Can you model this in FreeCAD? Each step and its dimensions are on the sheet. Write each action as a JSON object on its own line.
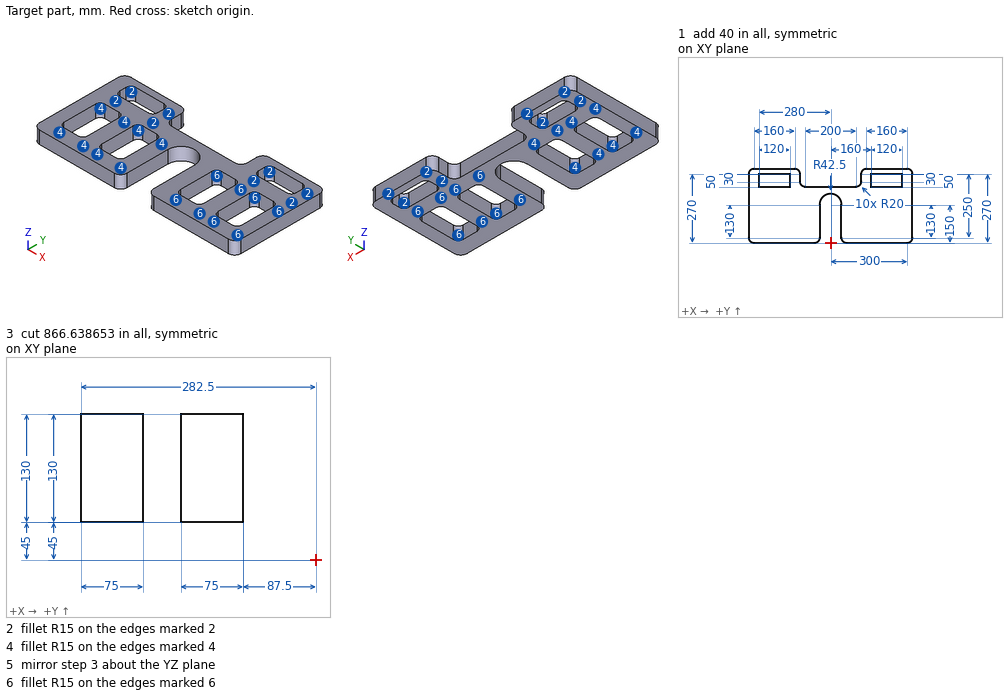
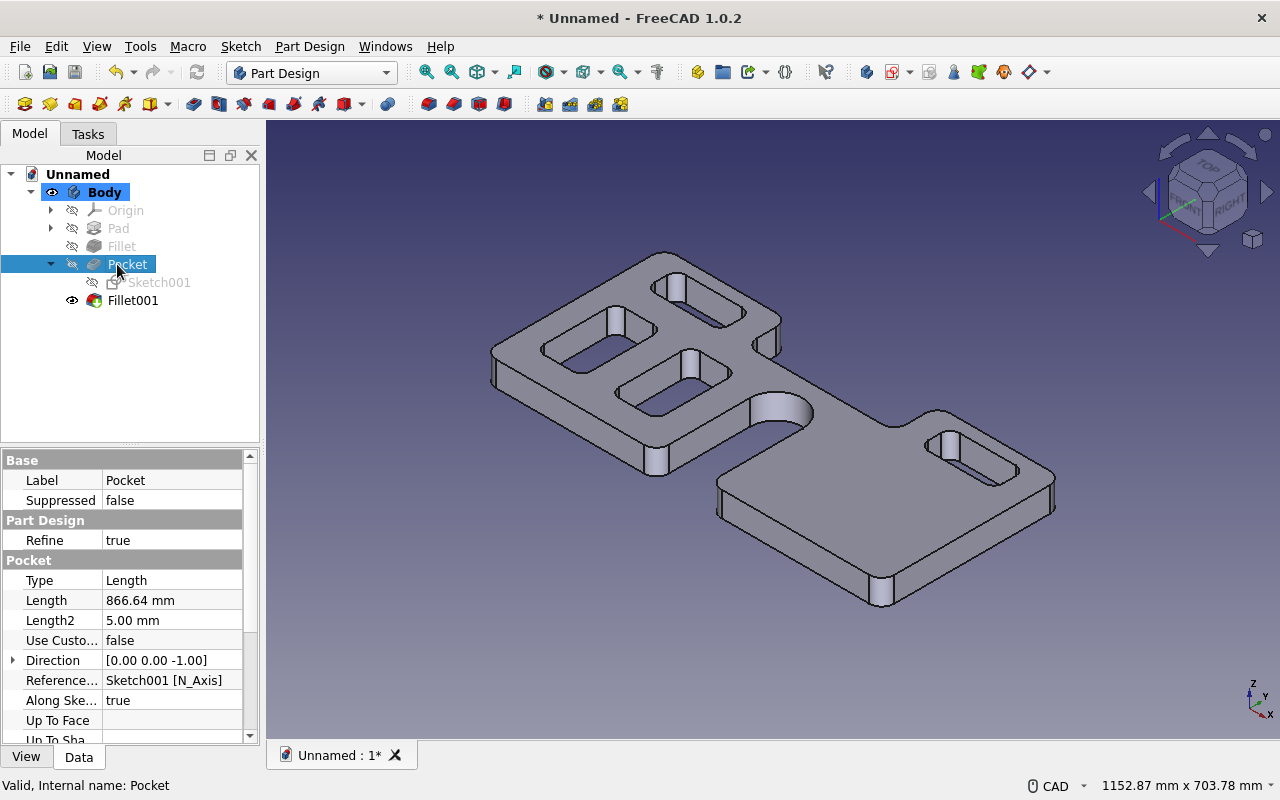
{"action": "left_click", "coordinate": [545, 104]}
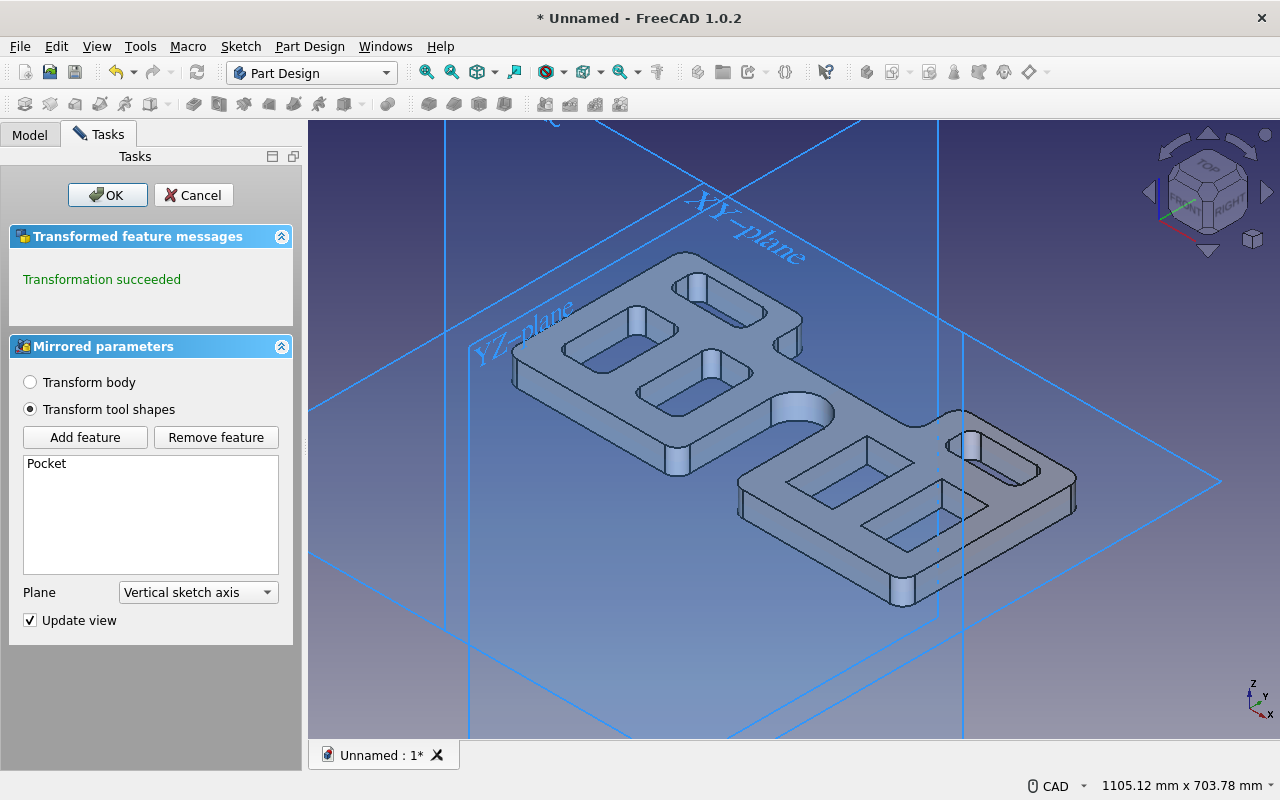
{"action": "left_click", "coordinate": [199, 592]}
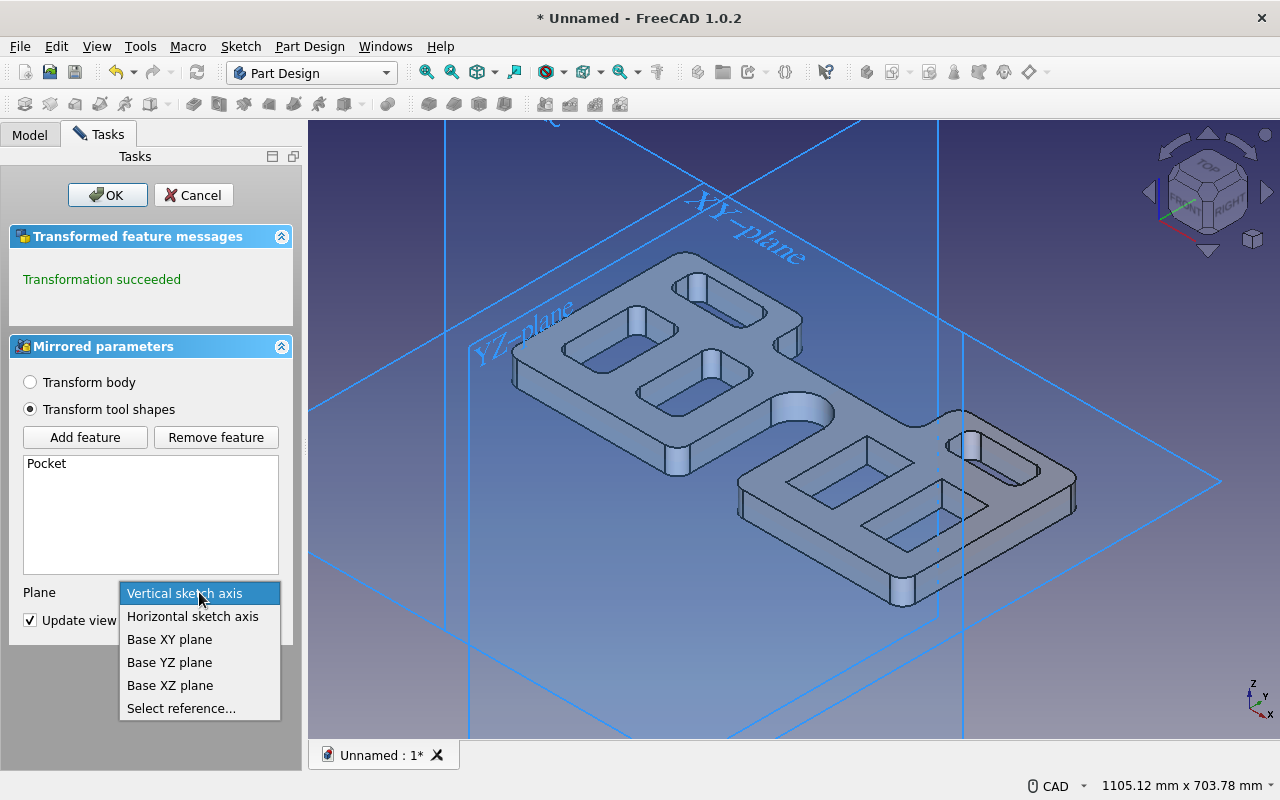
{"action": "left_click", "coordinate": [198, 662]}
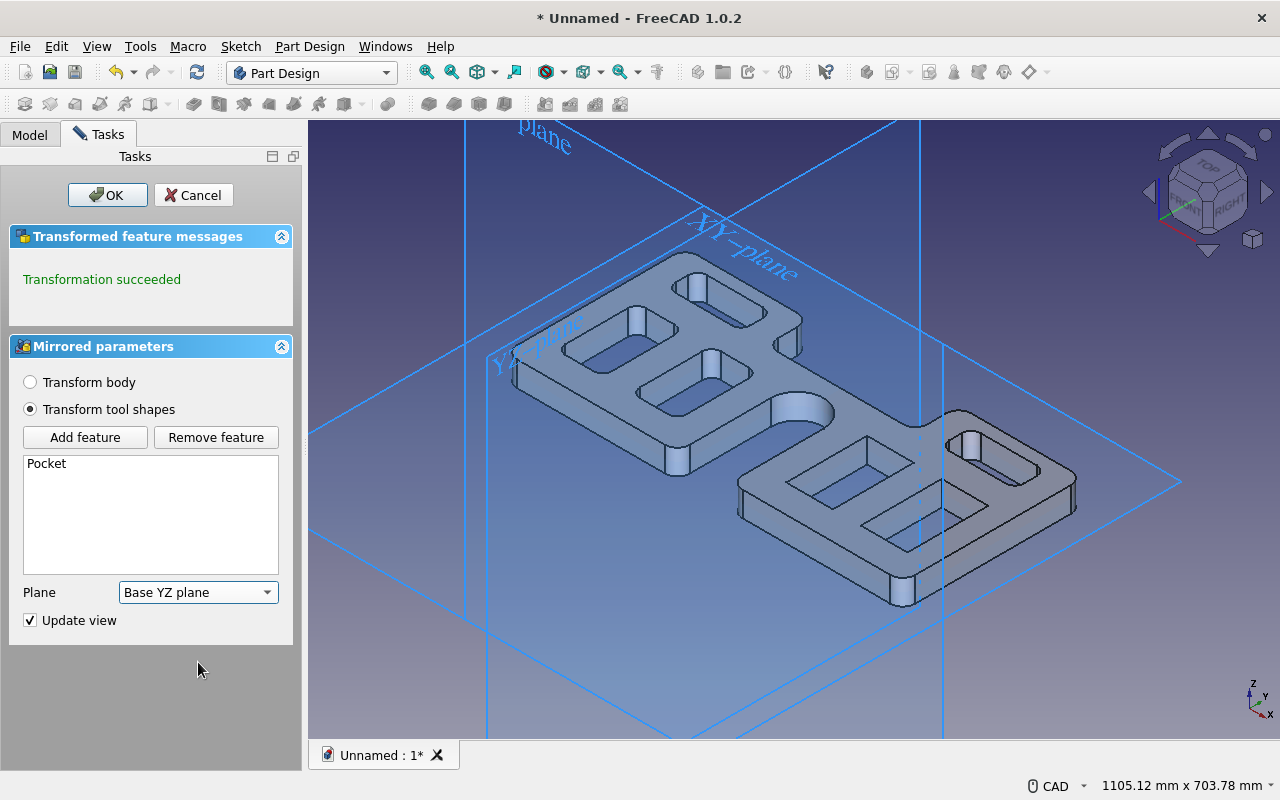
{"action": "left_click", "coordinate": [108, 195]}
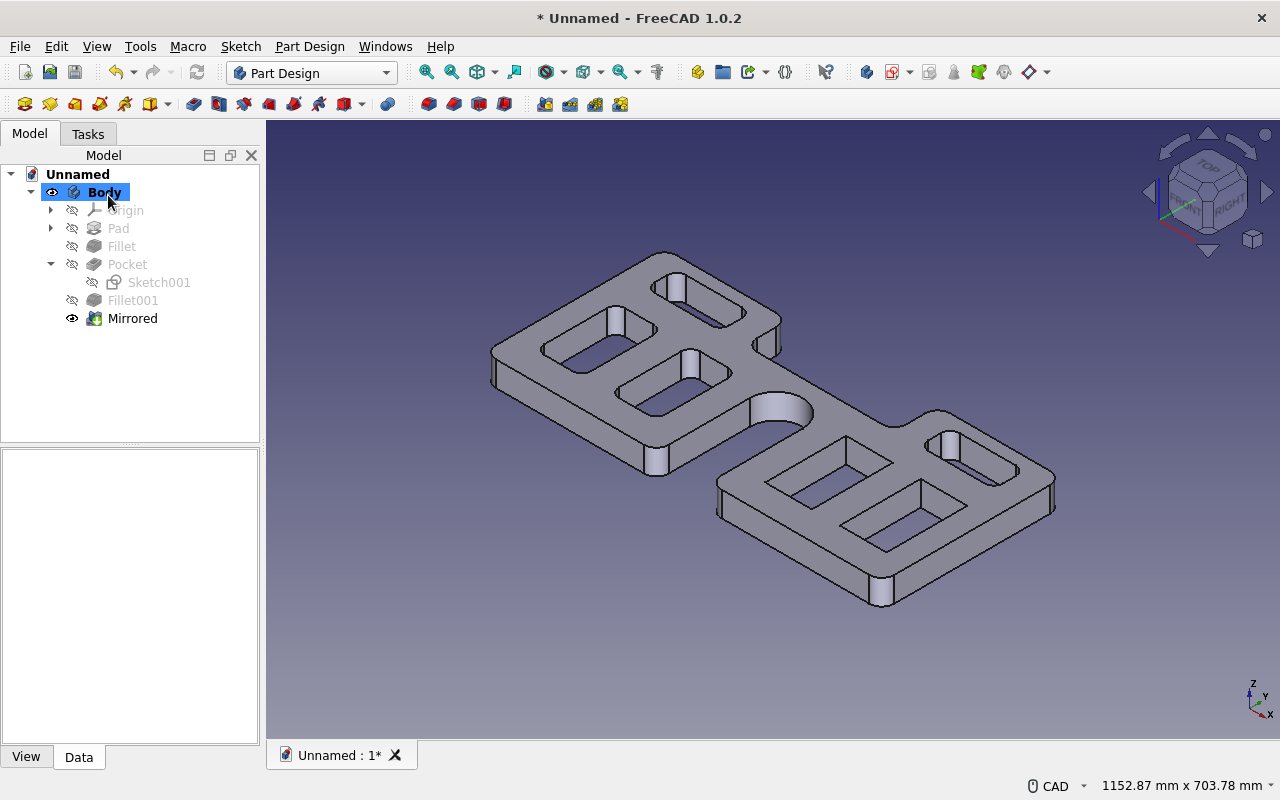
{"action": "key", "text": "2"}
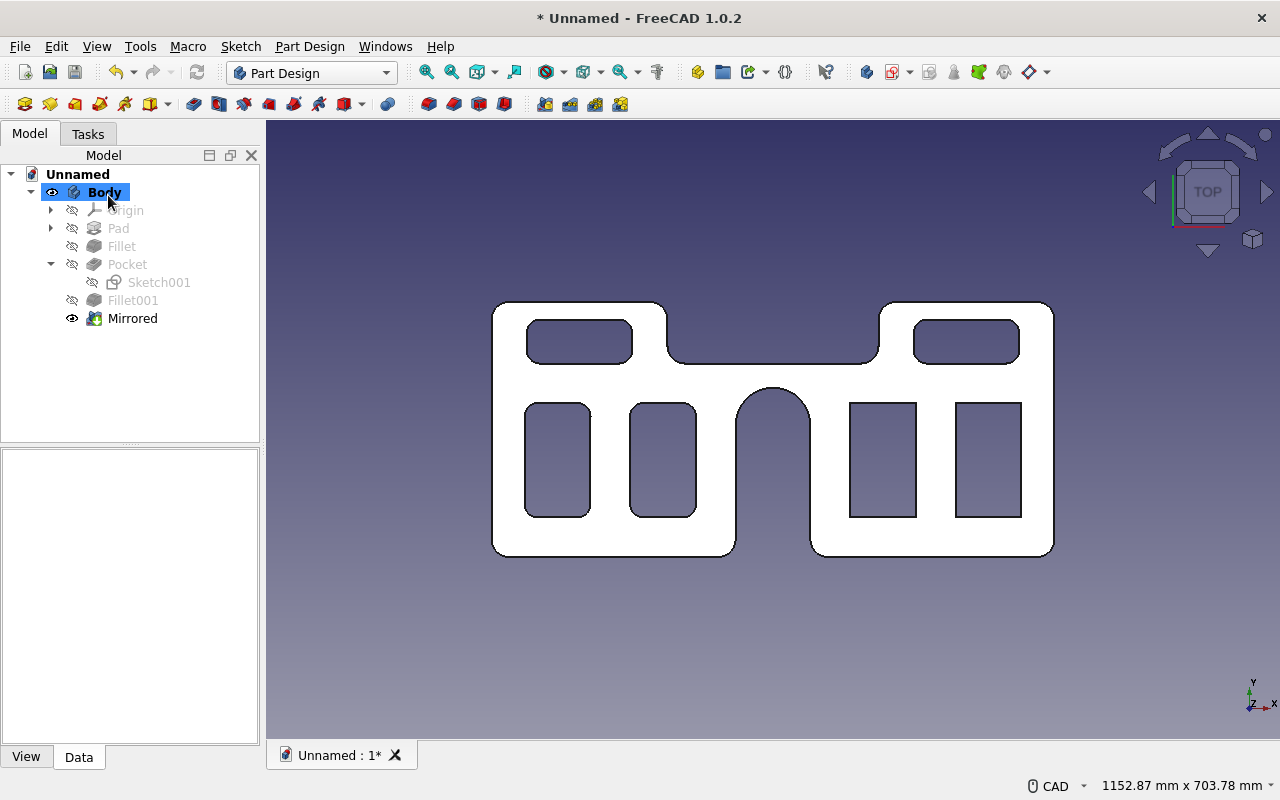
{"action": "key", "text": "0"}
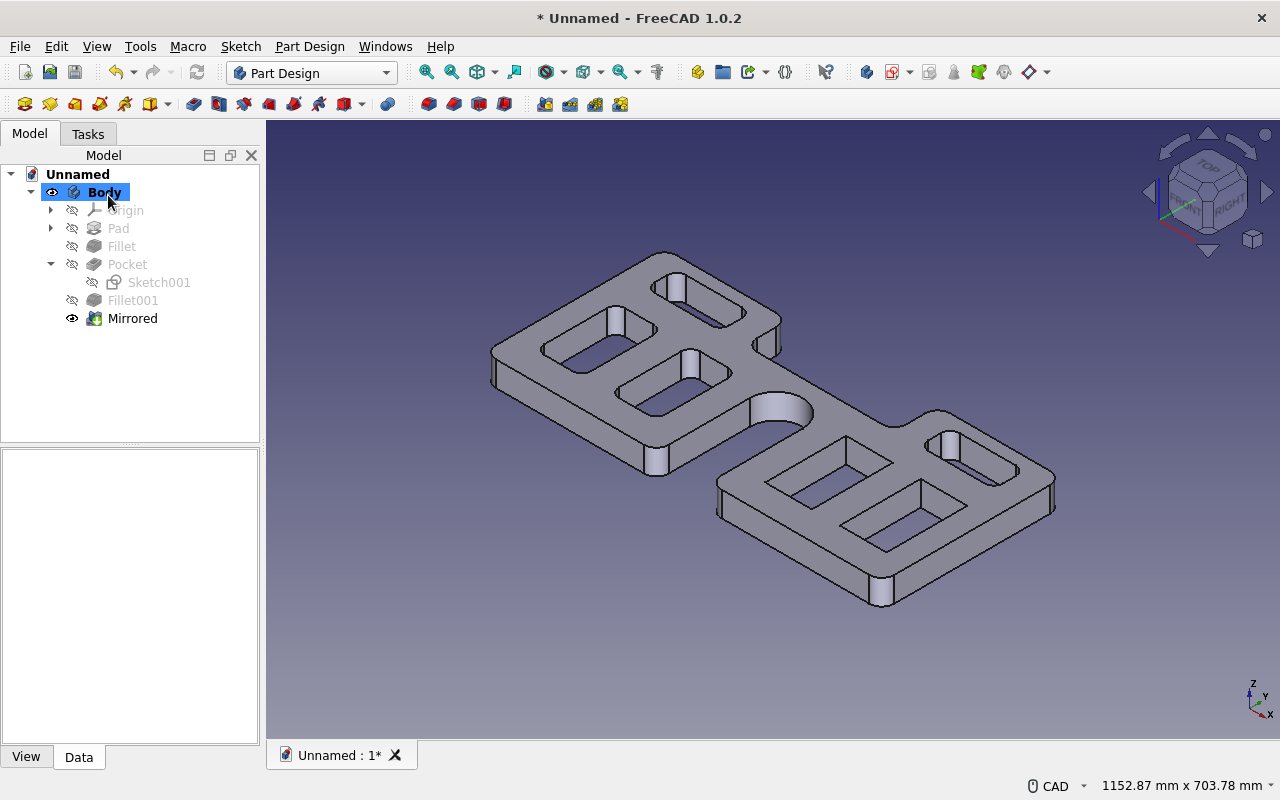
{"action": "key", "text": "1"}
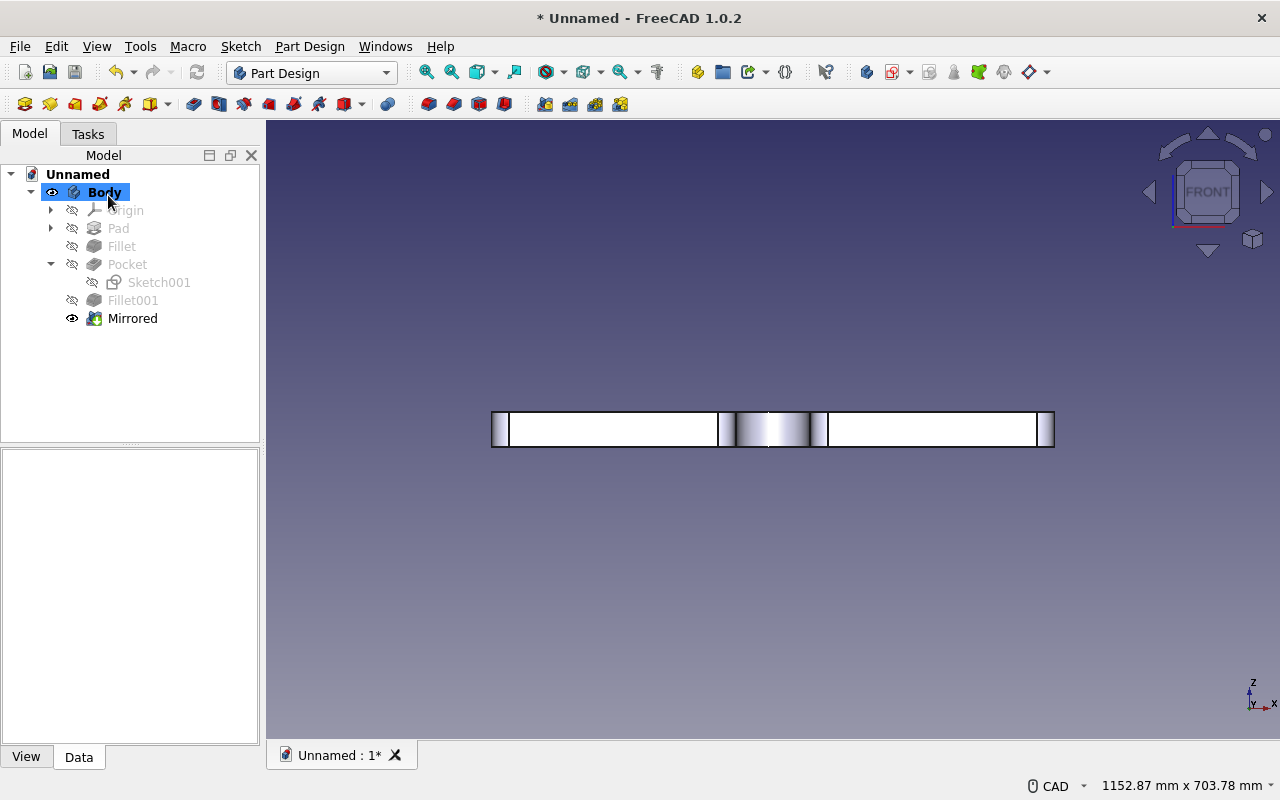
{"action": "key", "text": "3"}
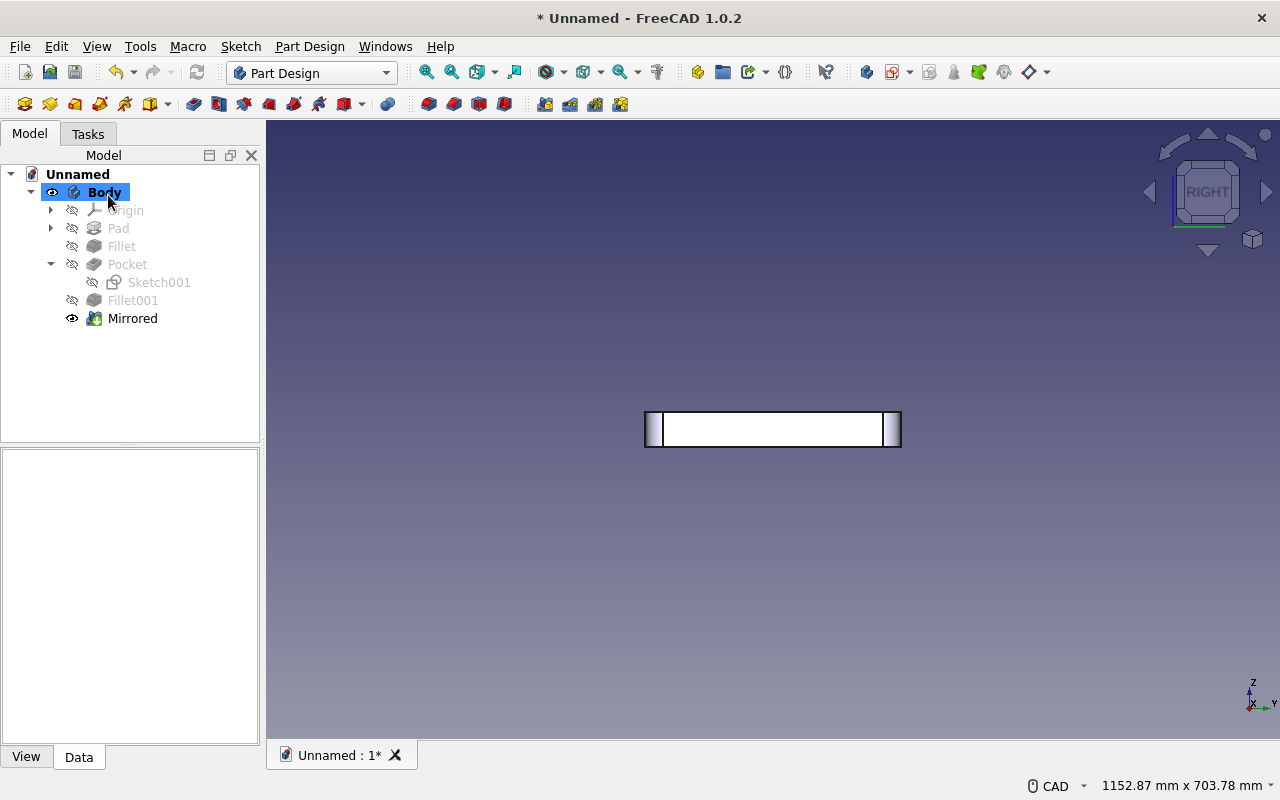
{"action": "key", "text": "v f"}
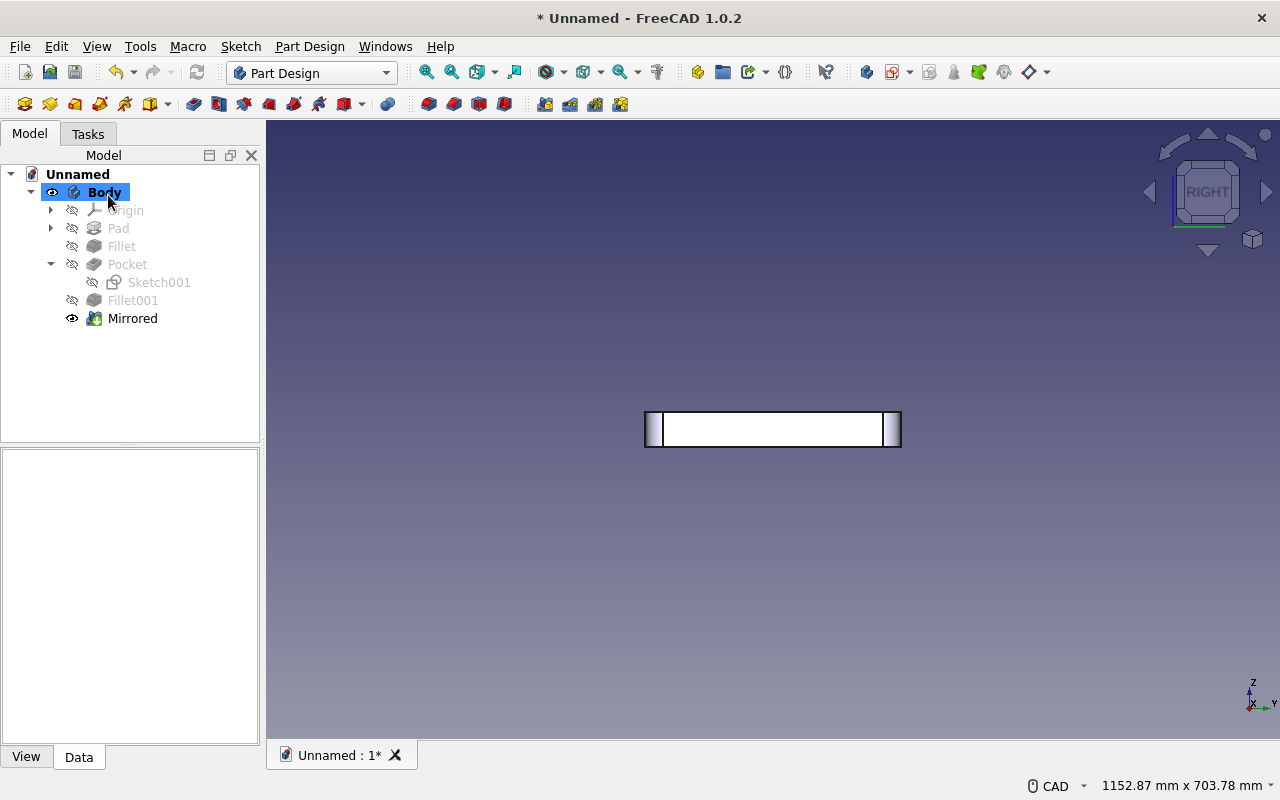
{"action": "key", "text": "5"}